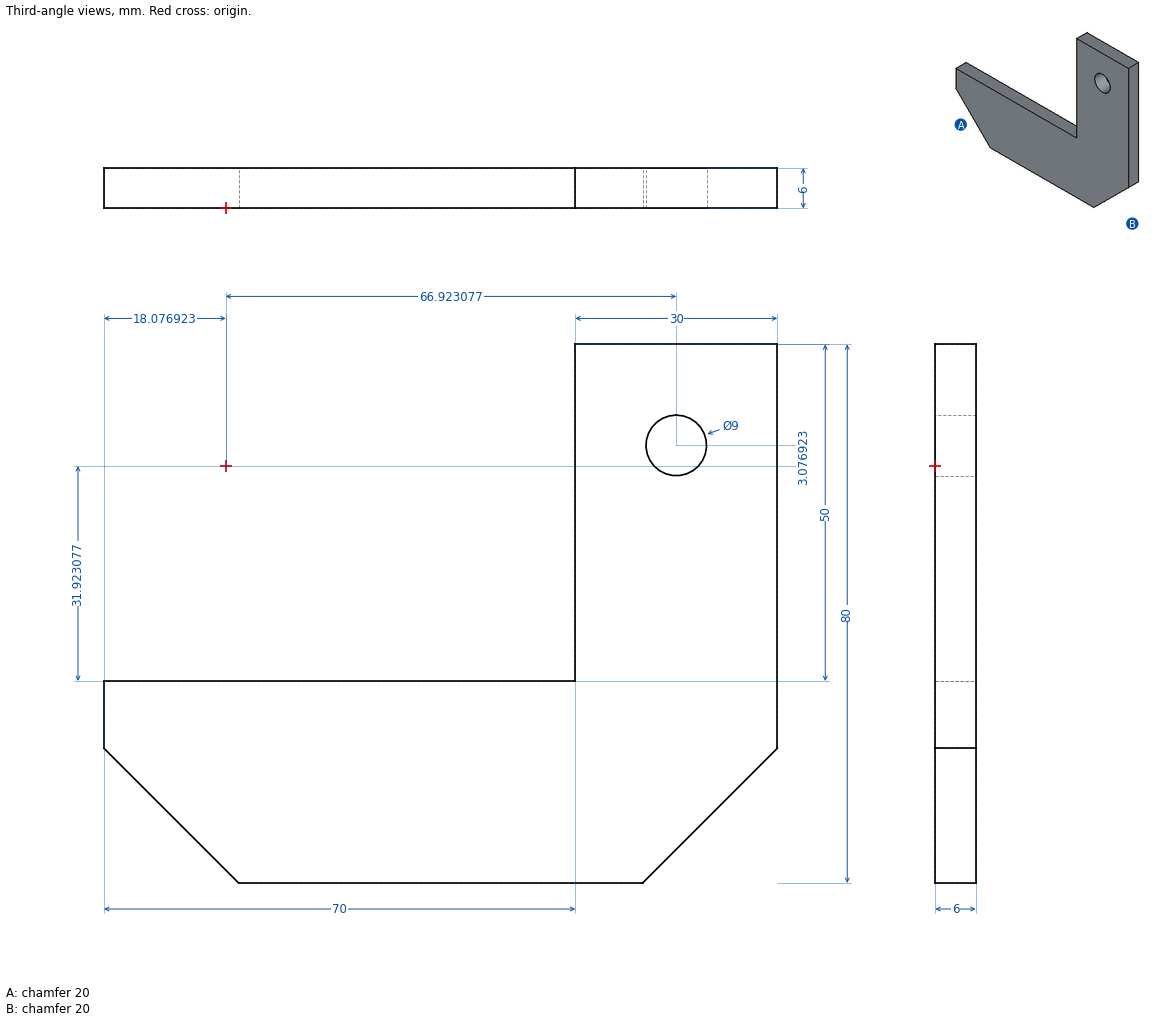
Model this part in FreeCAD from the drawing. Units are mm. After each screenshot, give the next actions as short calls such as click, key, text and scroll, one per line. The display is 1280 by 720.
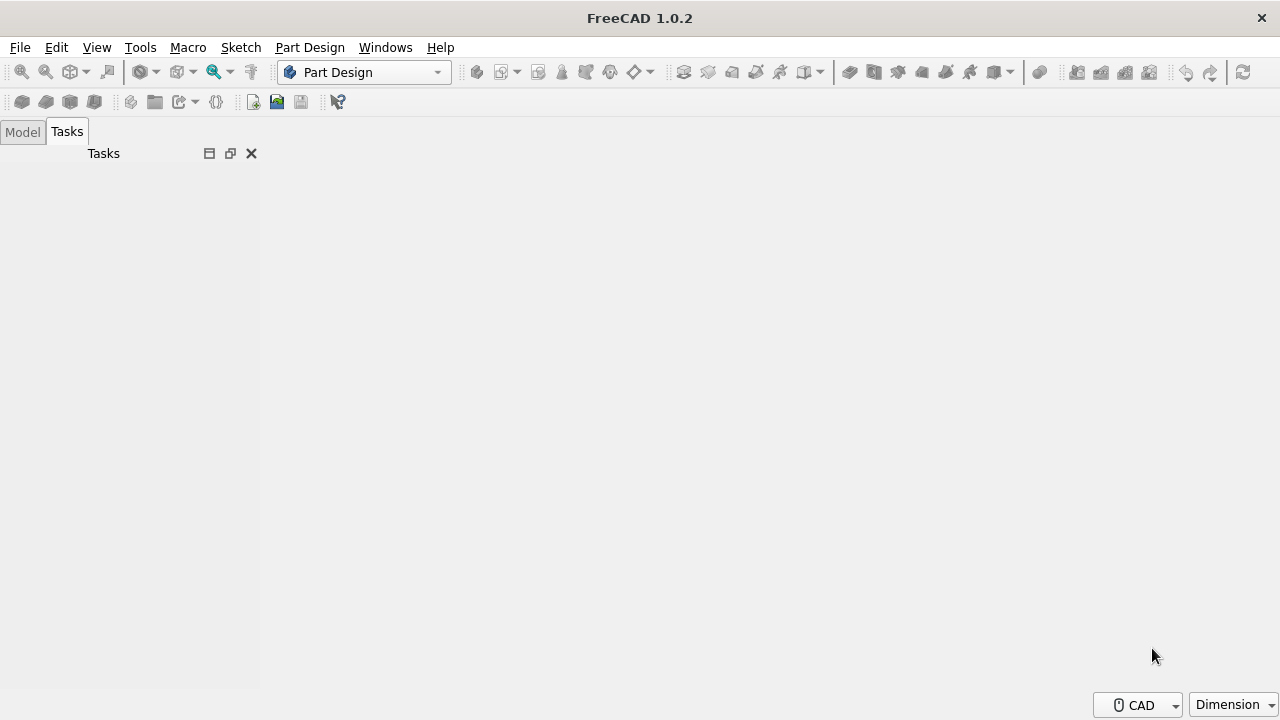
click(254, 102)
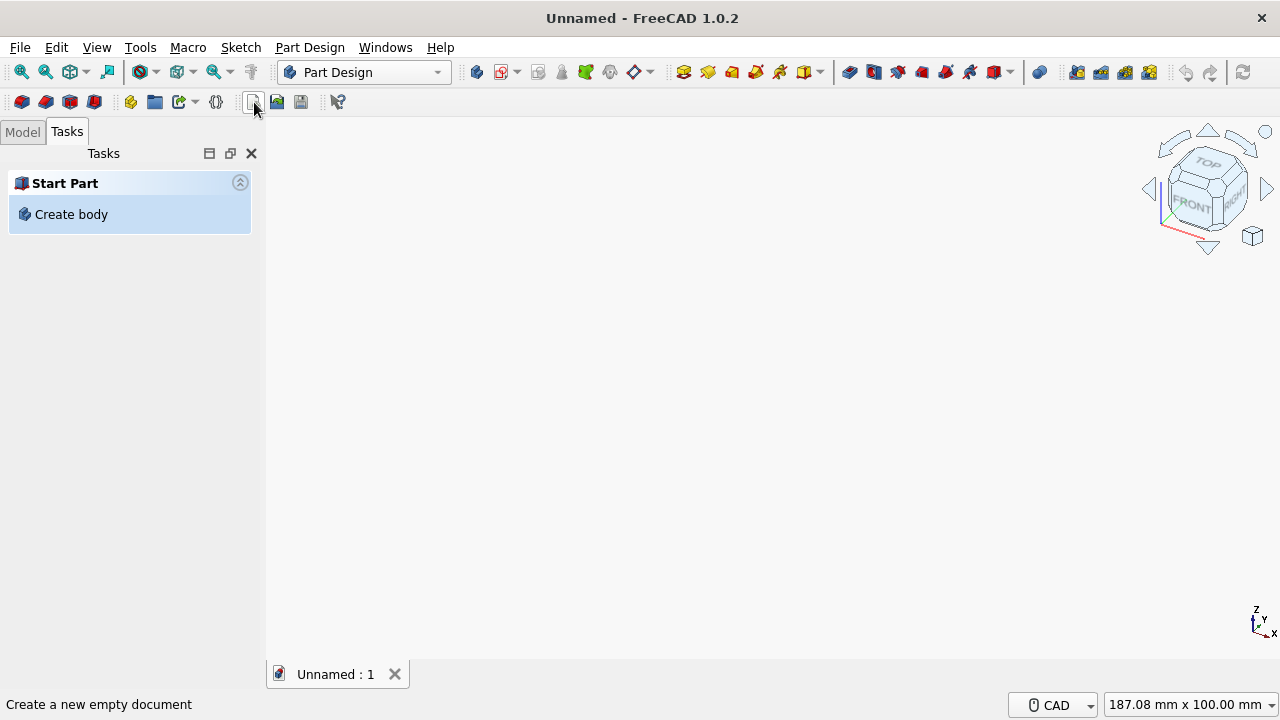
click(502, 72)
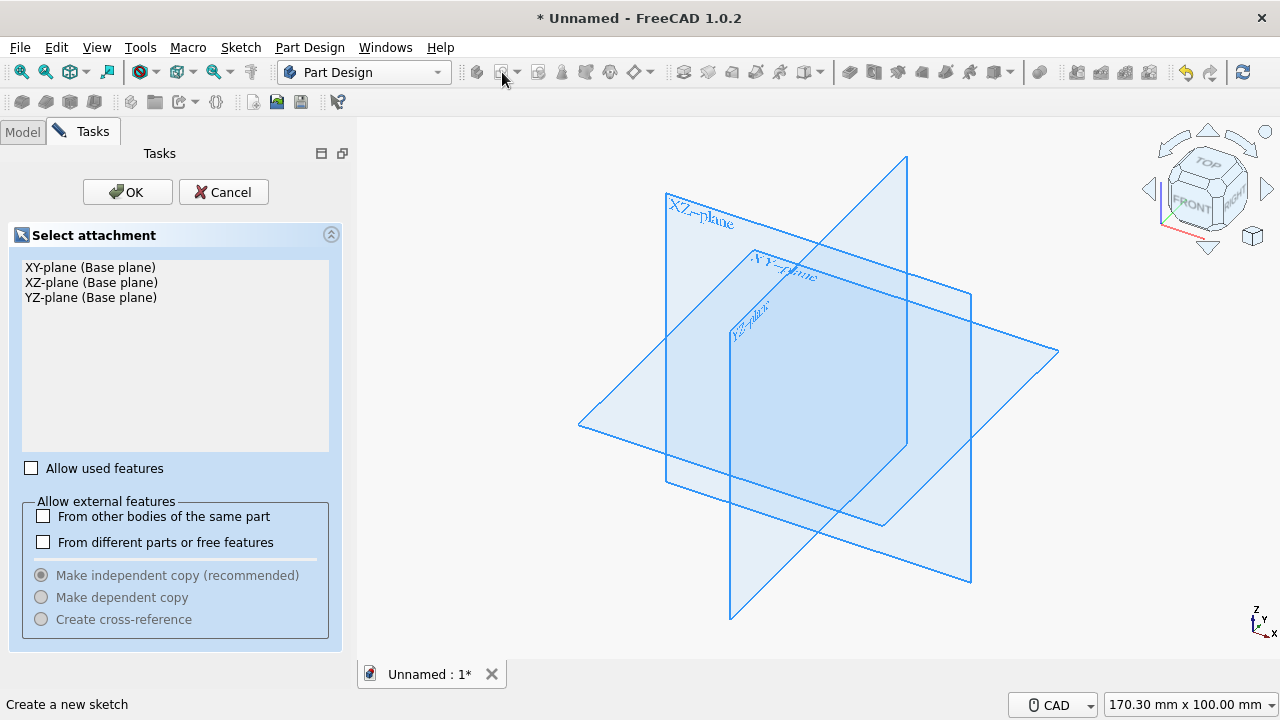
click(82, 282)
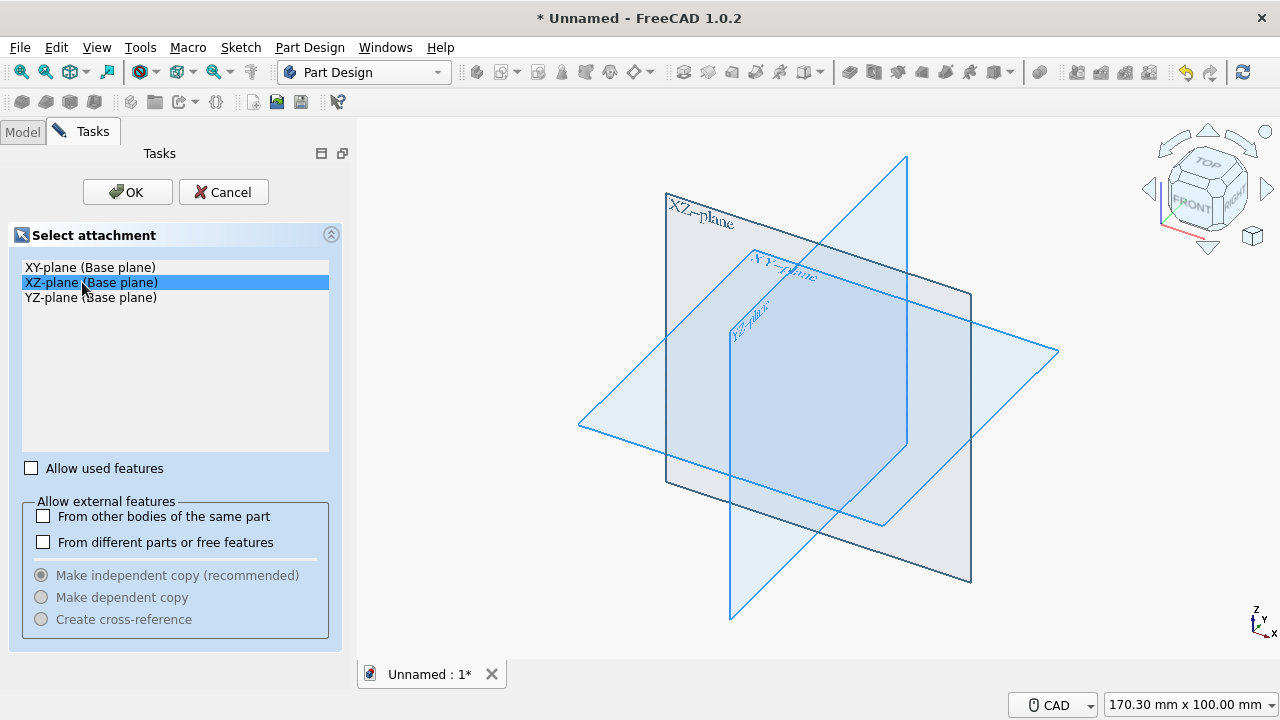
click(128, 192)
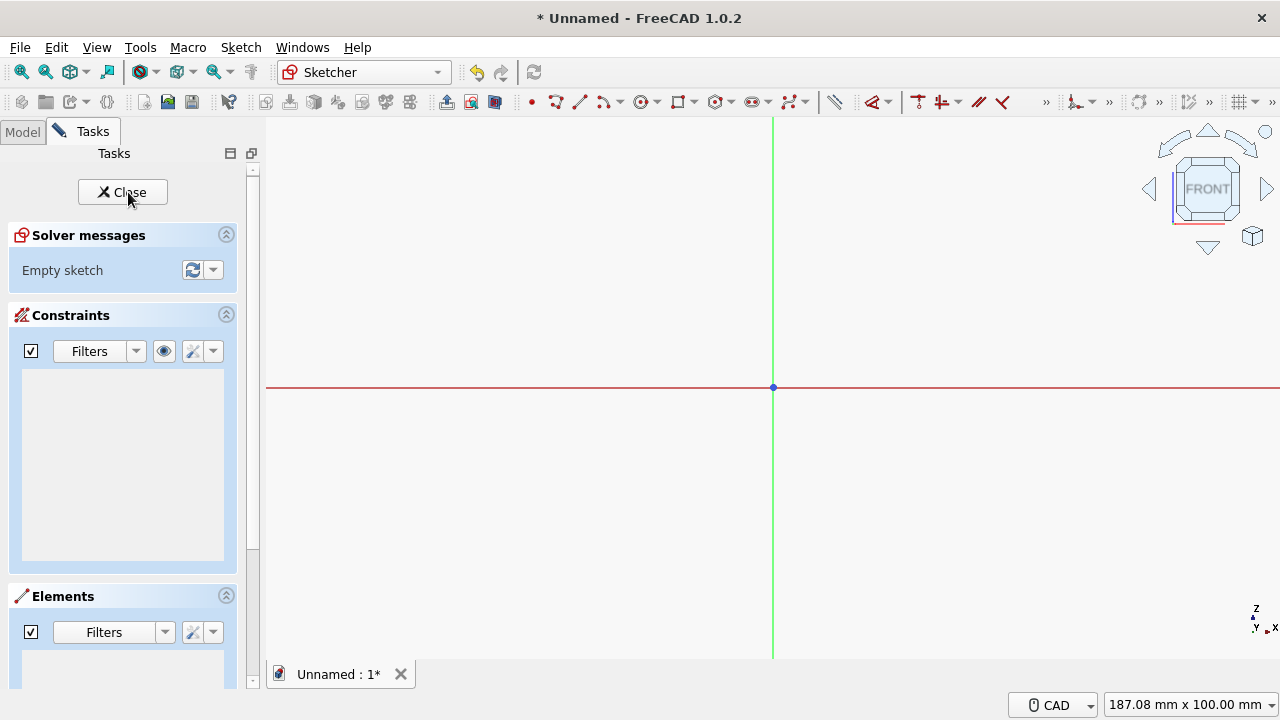
scroll(294, 146, down, 2)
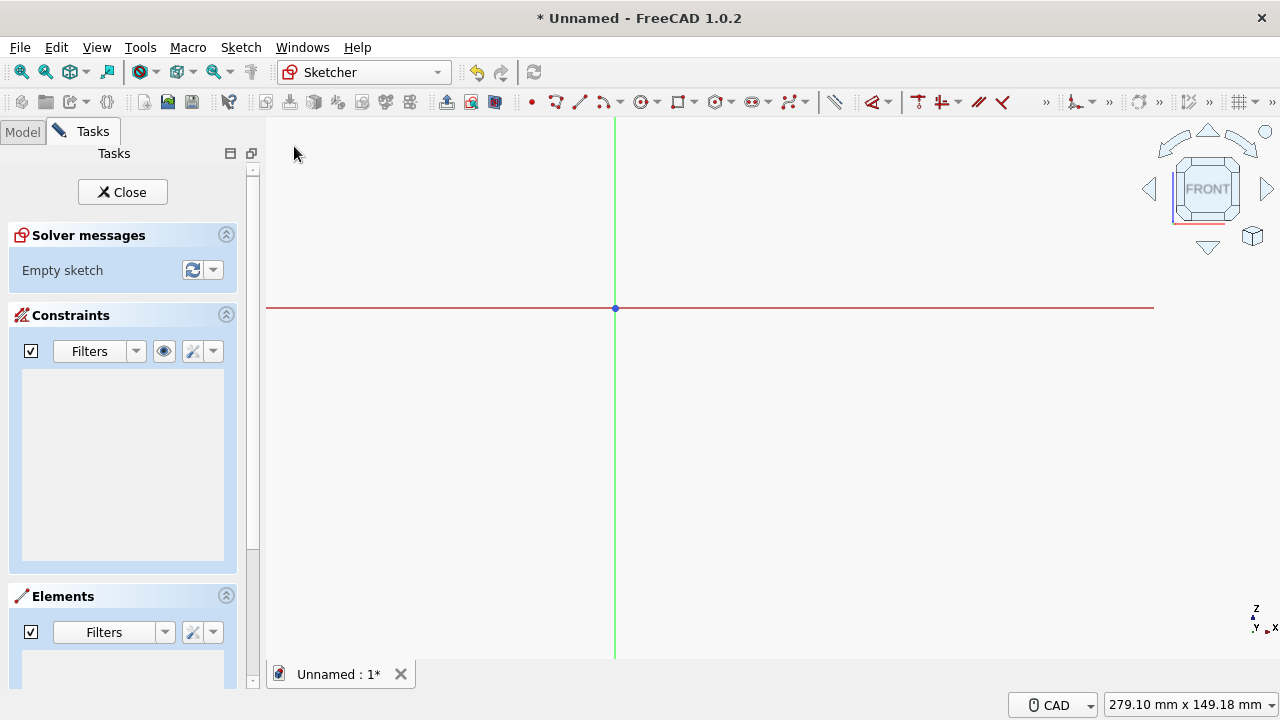
key(g)
key(m)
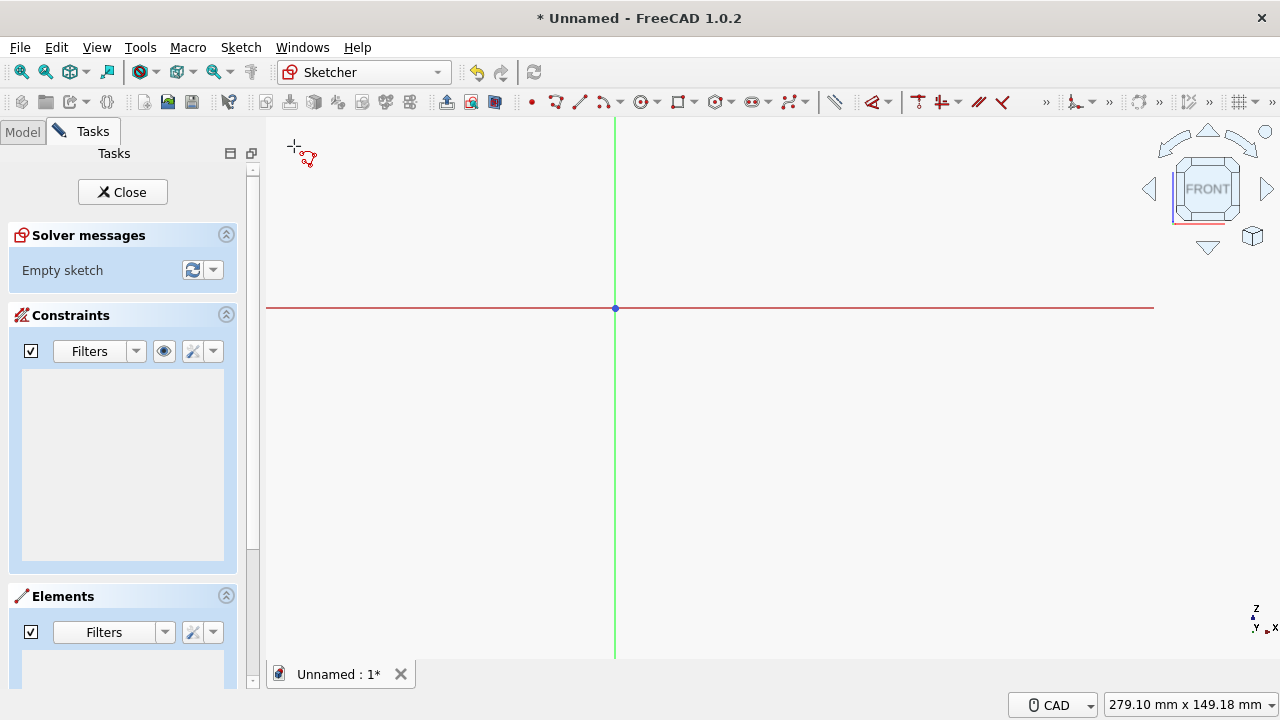
click(549, 424)
click(804, 424)
click(804, 243)
click(913, 243)
click(913, 533)
click(549, 533)
click(549, 425)
key(Escape)
key(Escape)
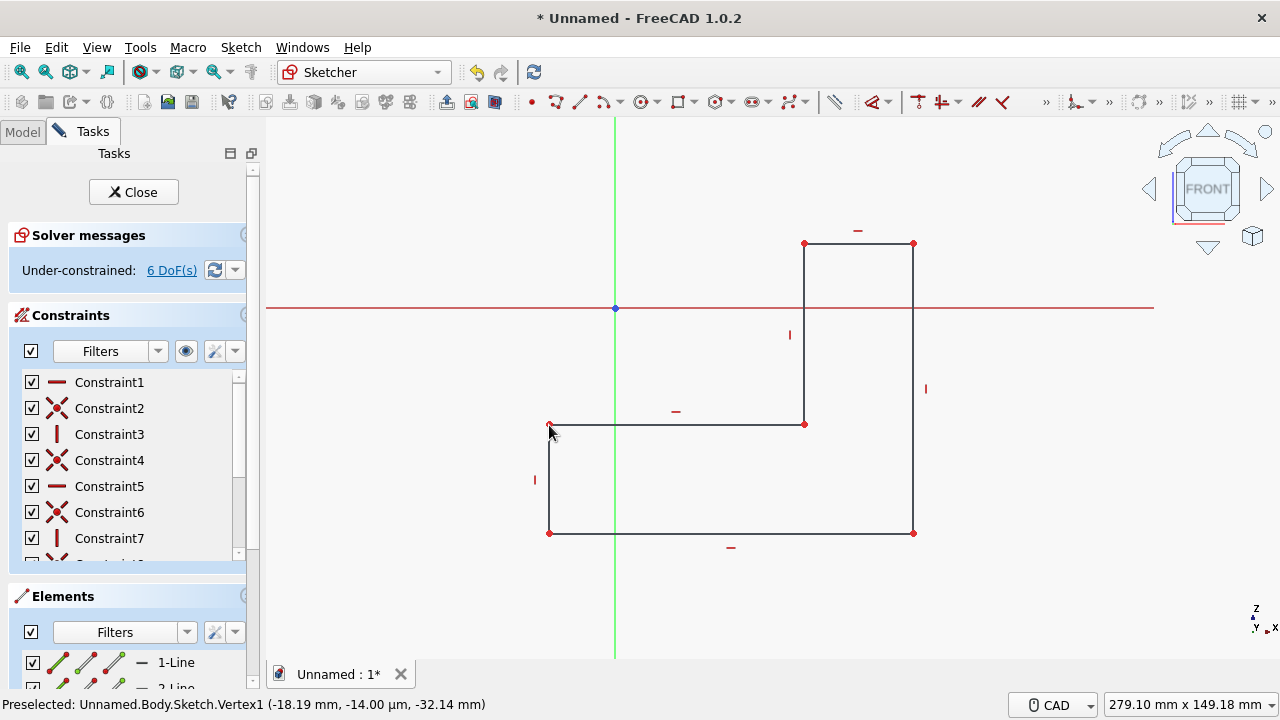
scroll(626, 425, up, 2)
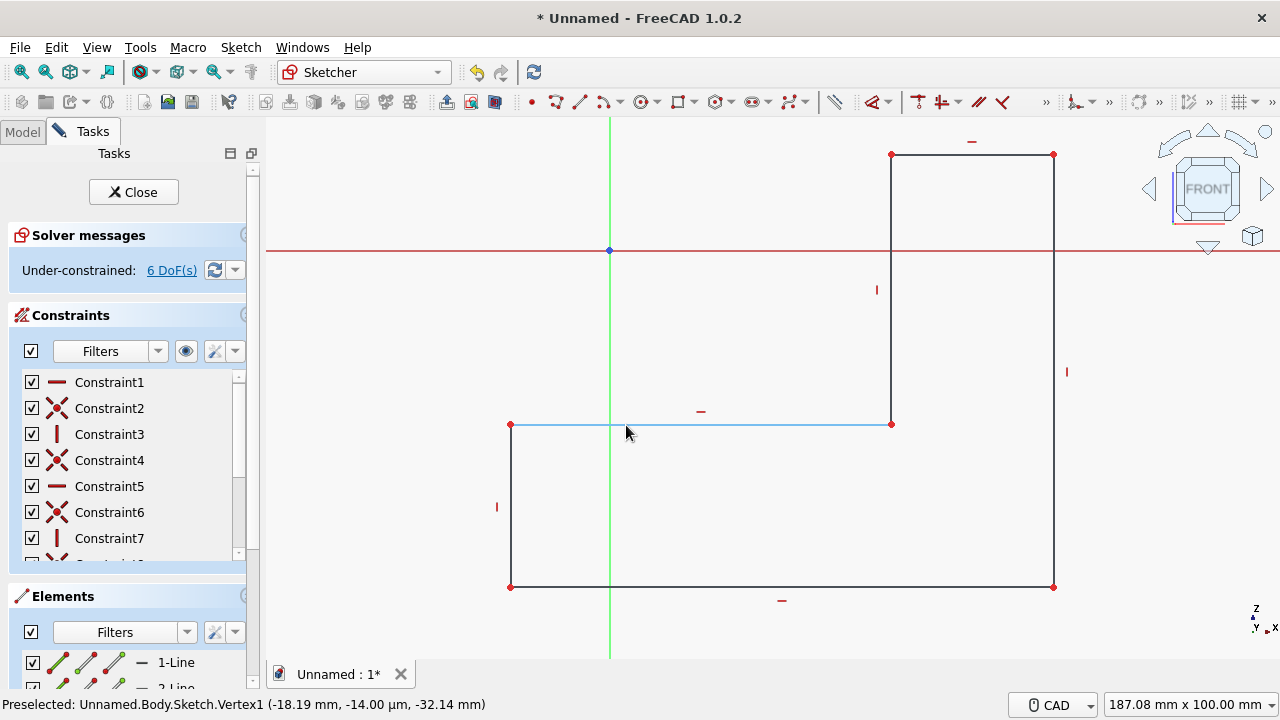
click(625, 425)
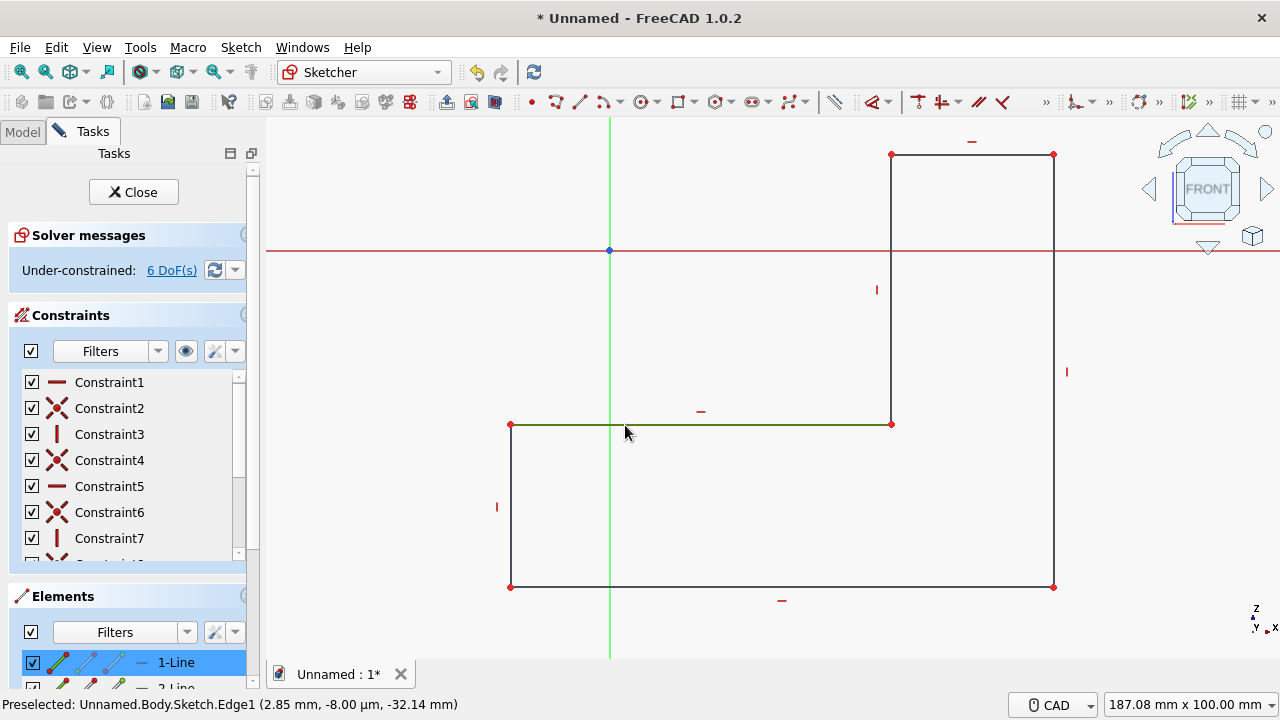
click(890, 102)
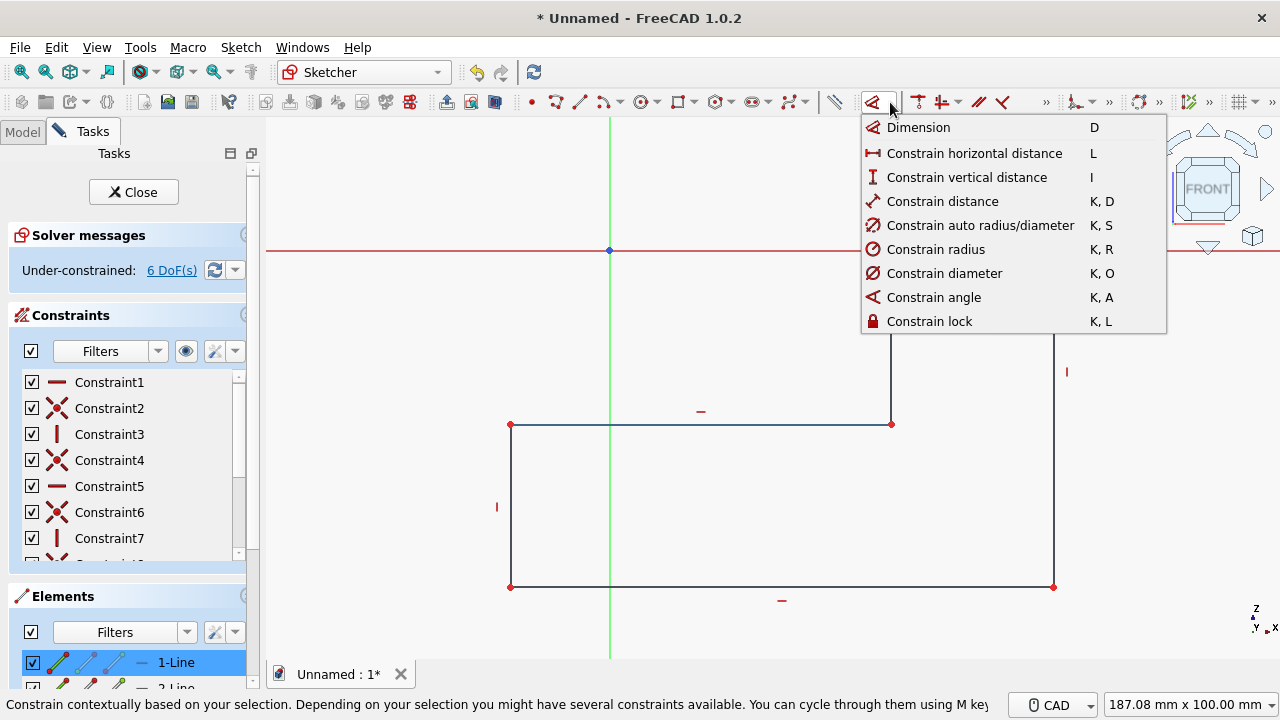
click(1014, 153)